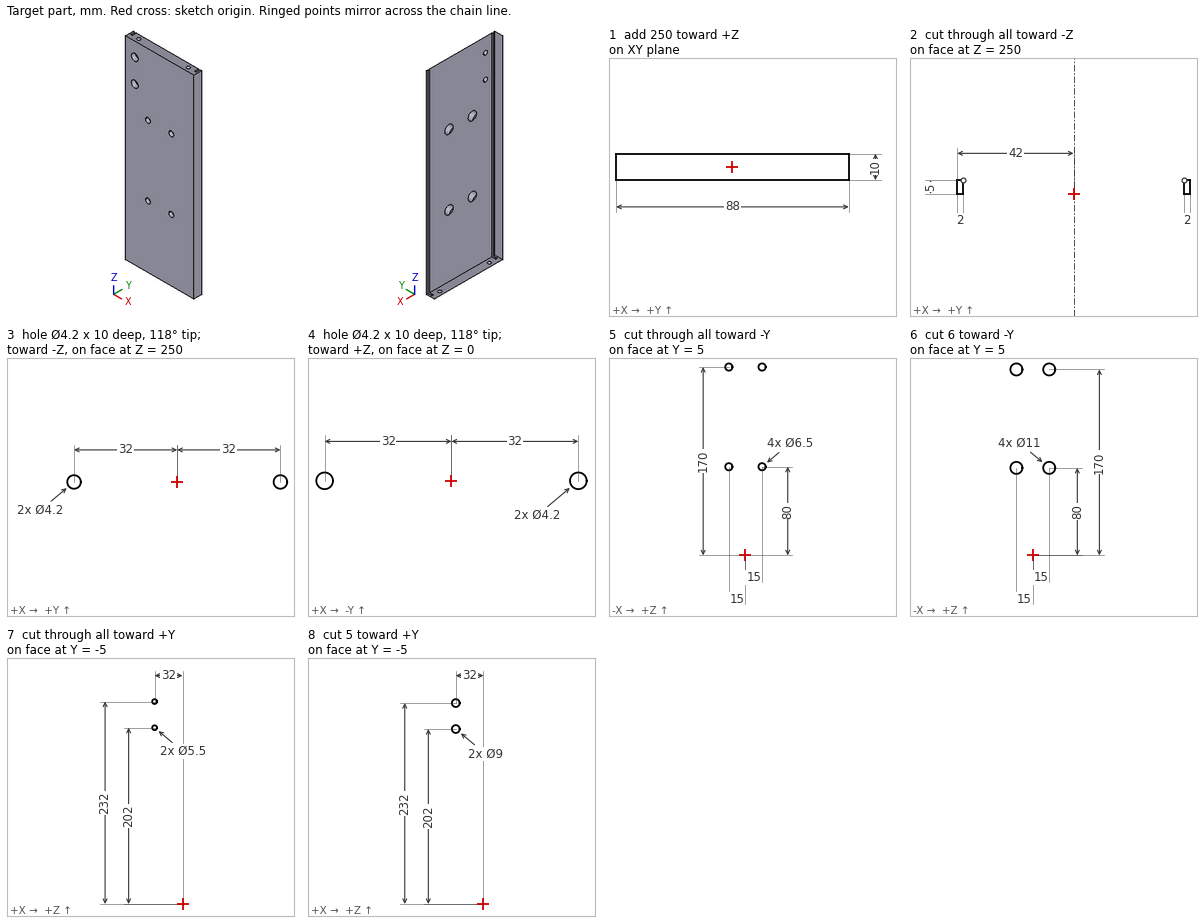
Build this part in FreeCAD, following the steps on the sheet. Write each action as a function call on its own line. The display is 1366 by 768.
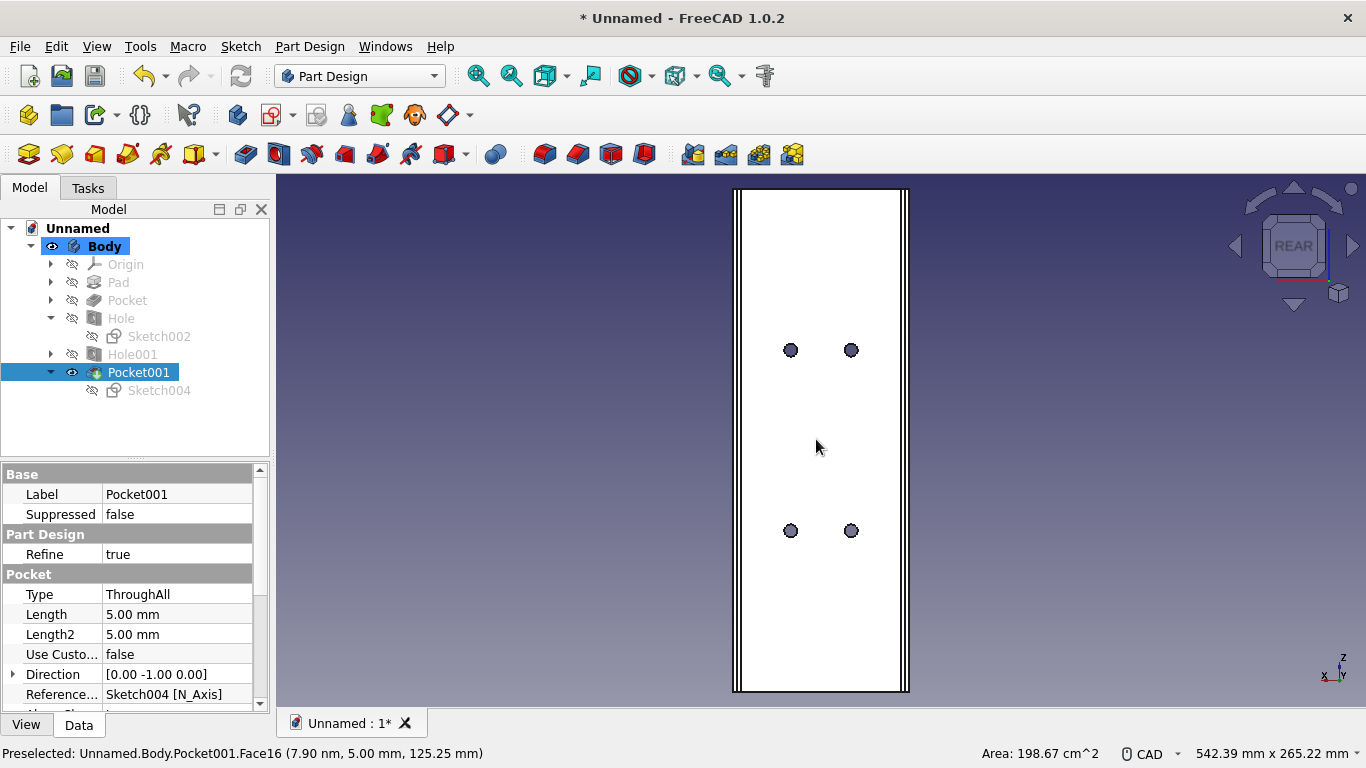
click(270, 116)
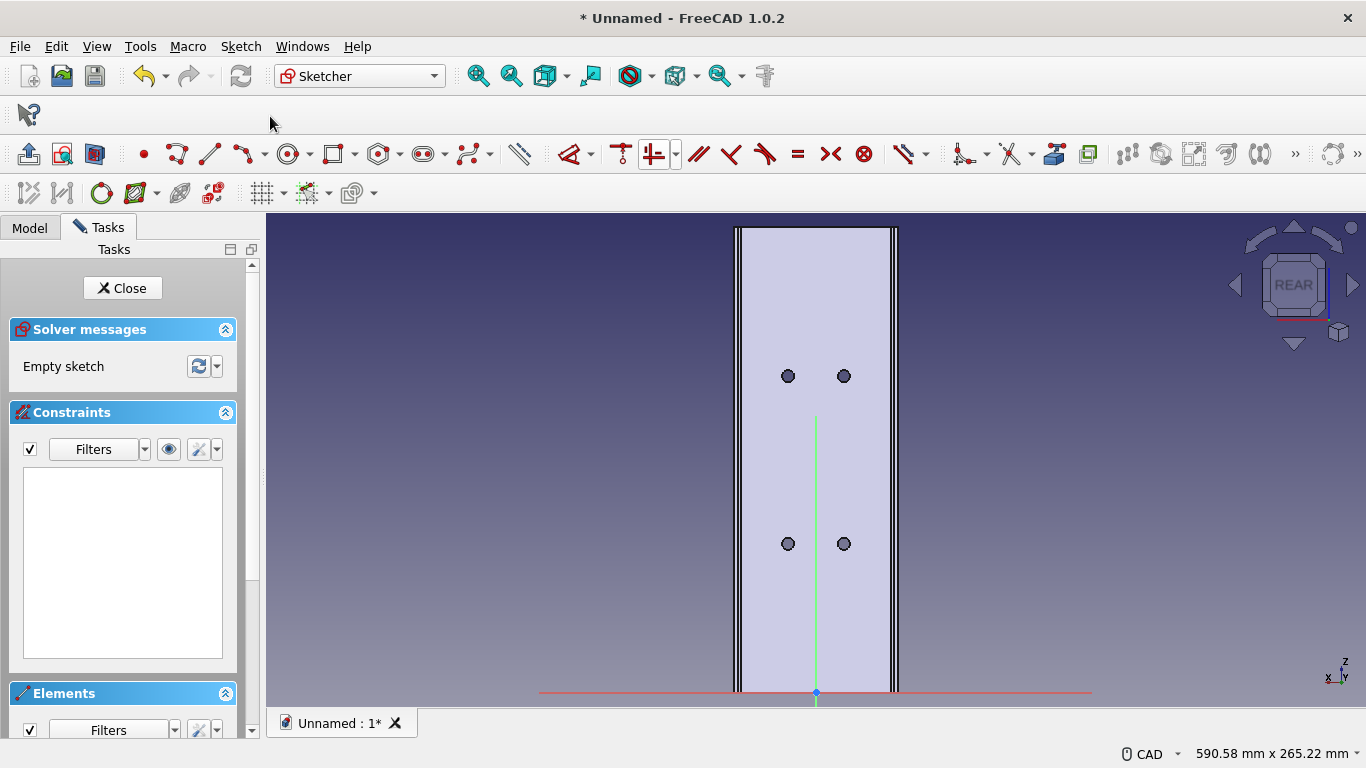
scroll(438, 241, down, 1)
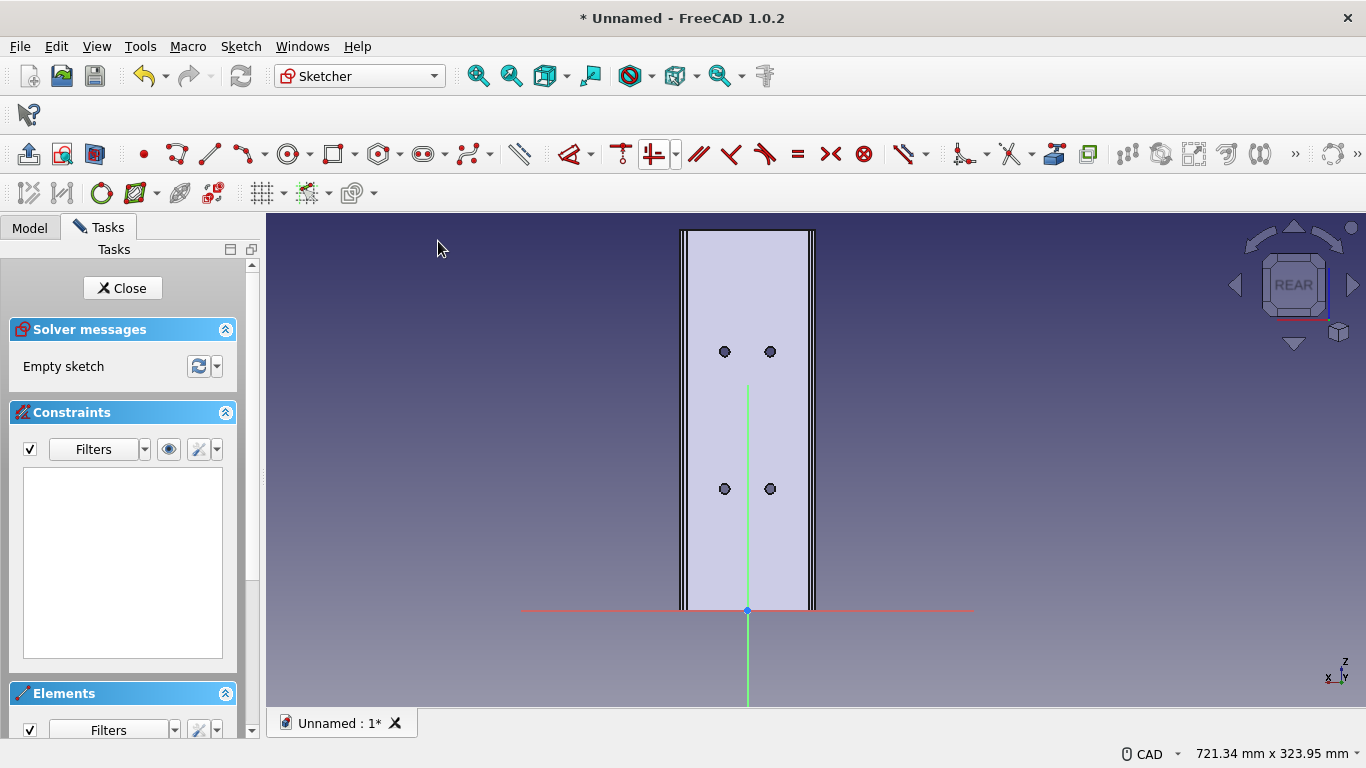
click(288, 154)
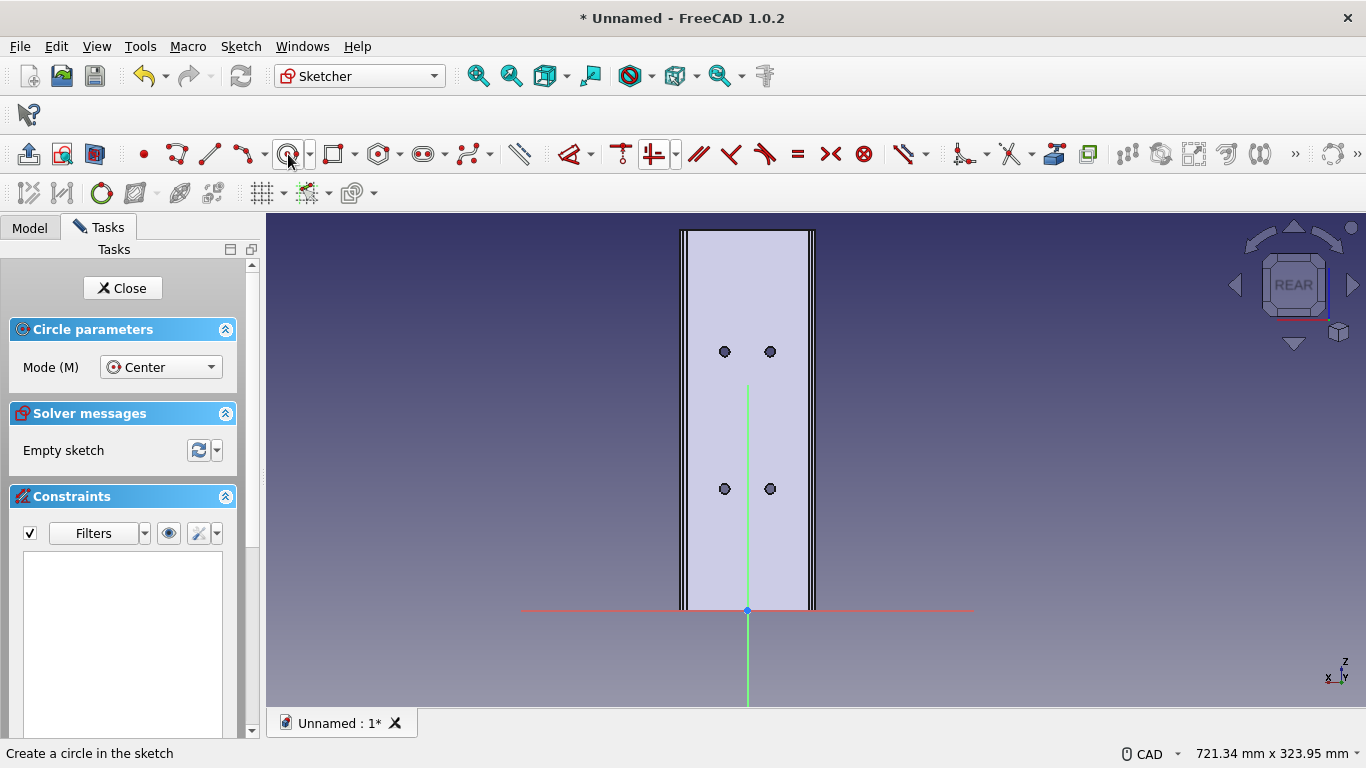
scroll(770, 489, up, 5)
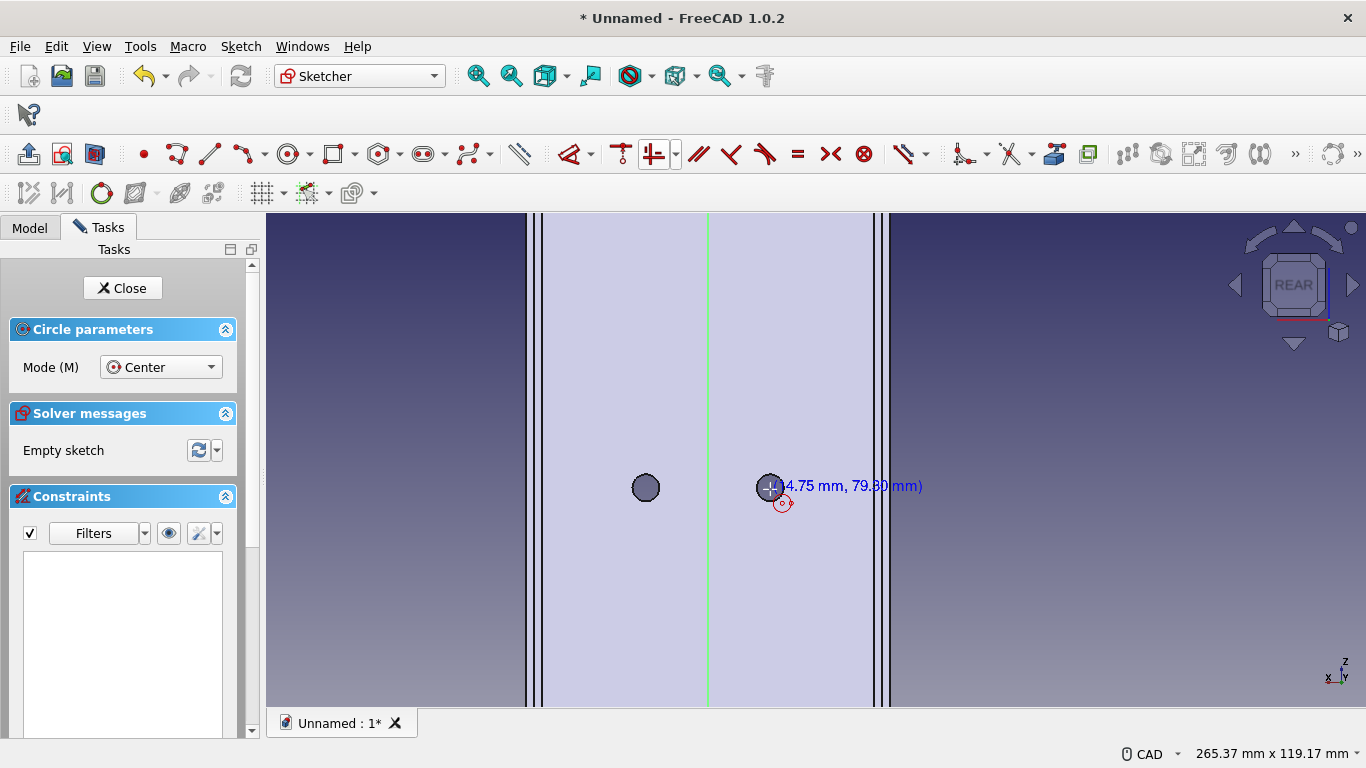
click(770, 488)
move(786, 472)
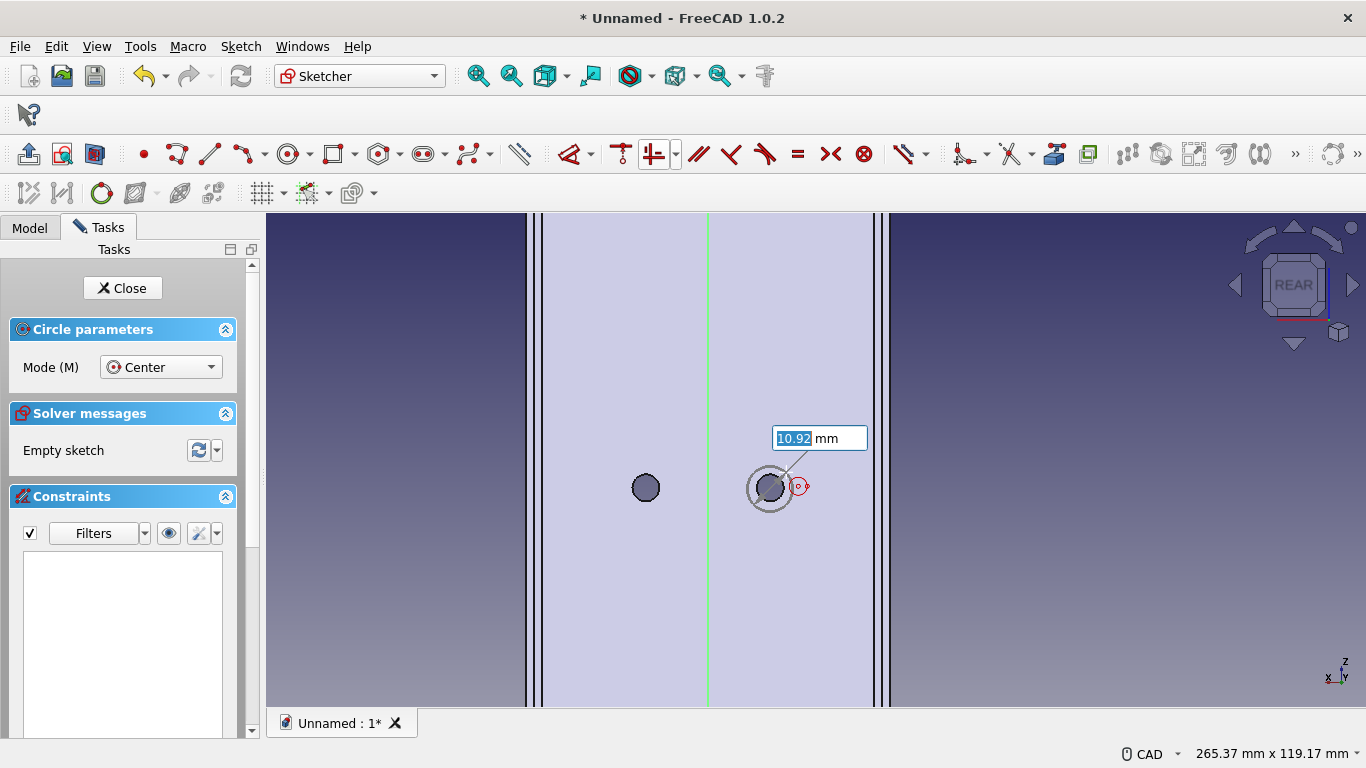
text(11)
key(Return)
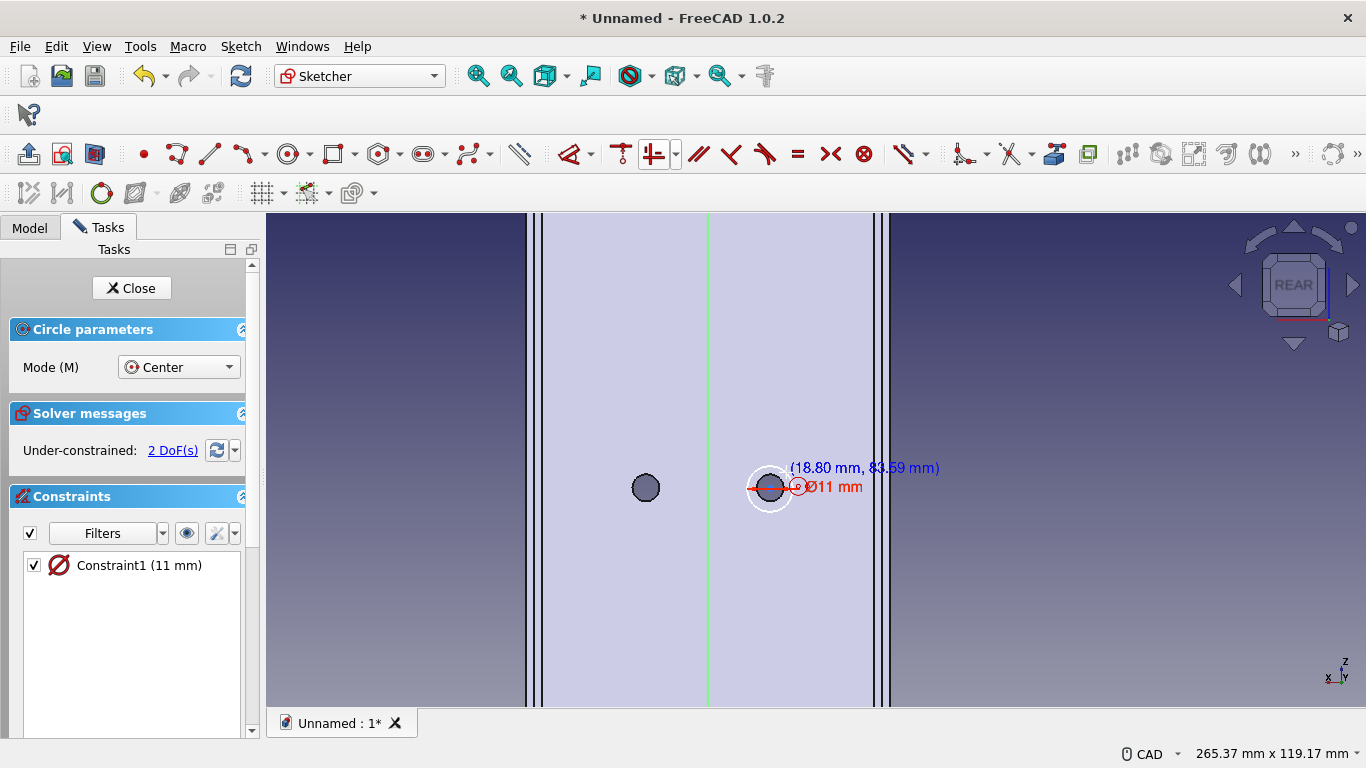
click(646, 488)
move(662, 472)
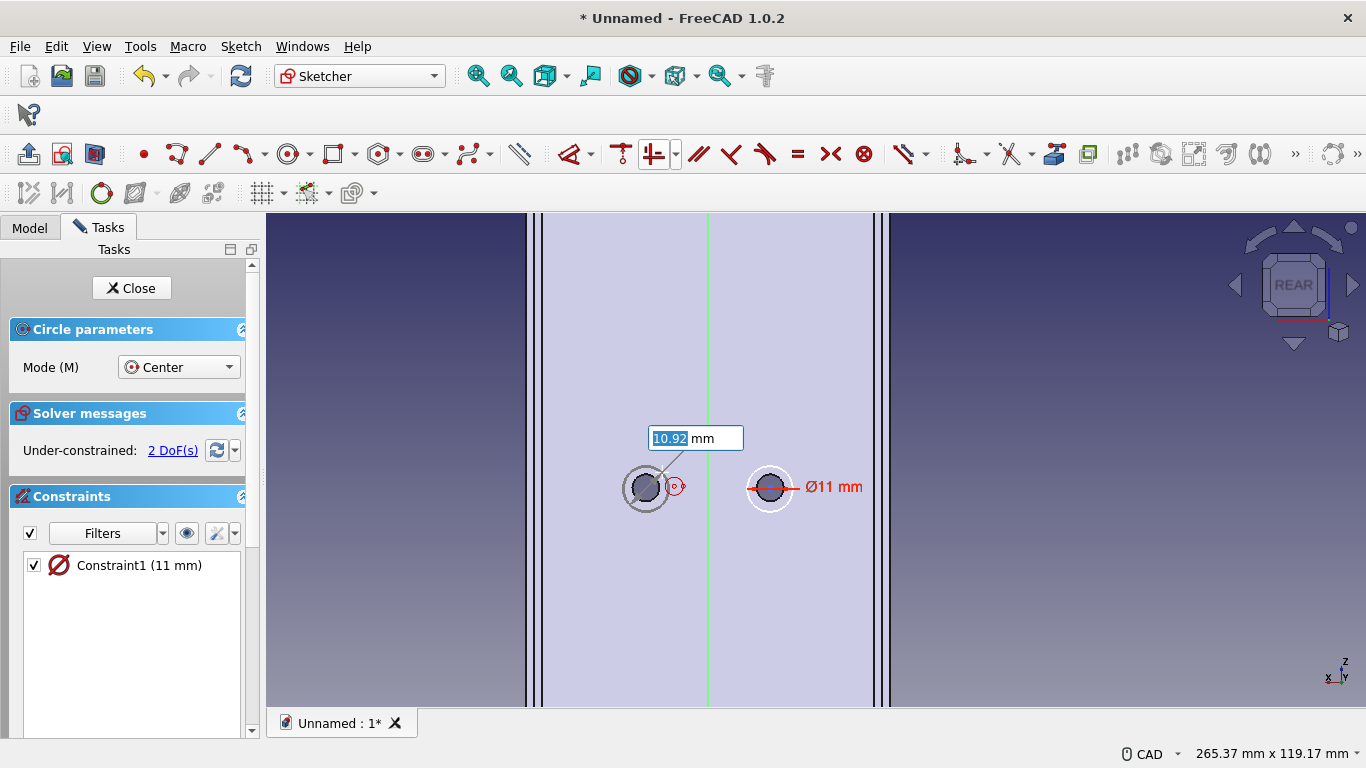
text(11)
key(Return)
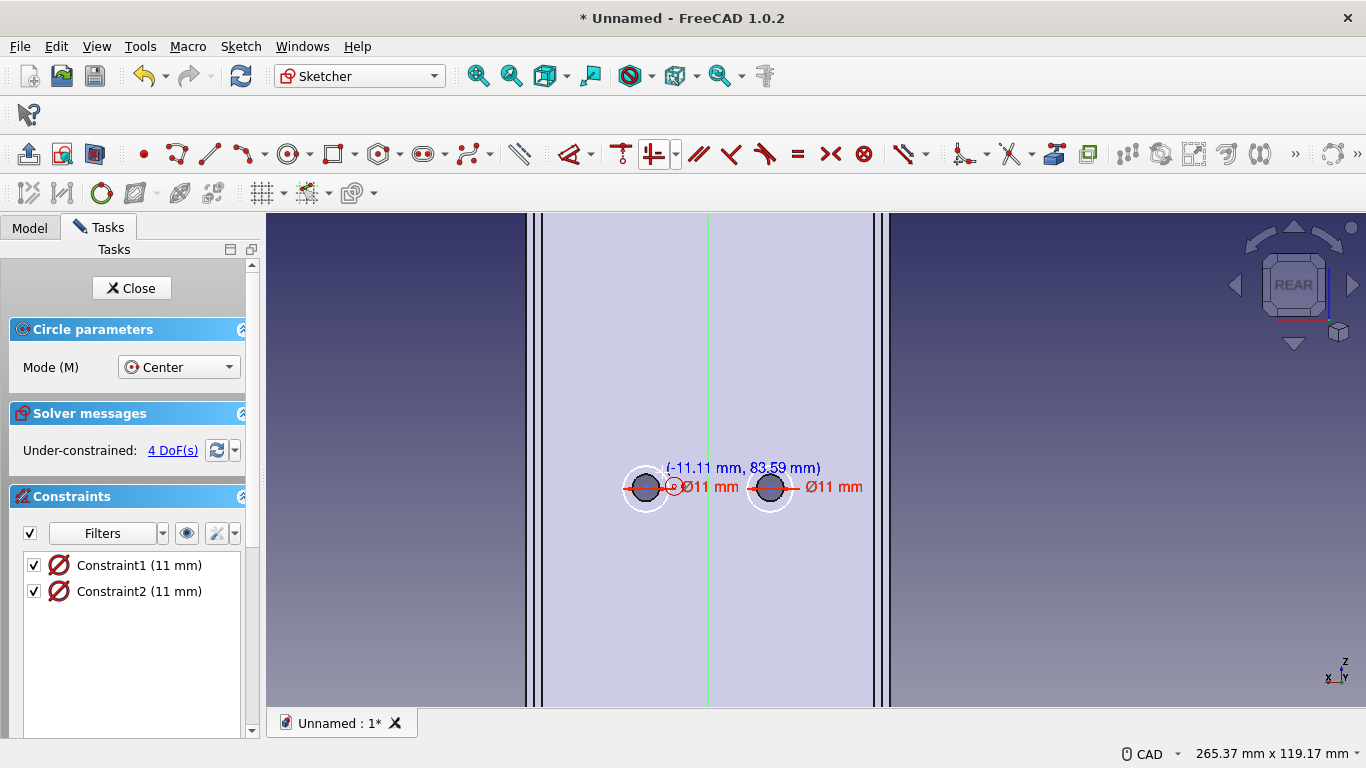
scroll(780, 463, down, 4)